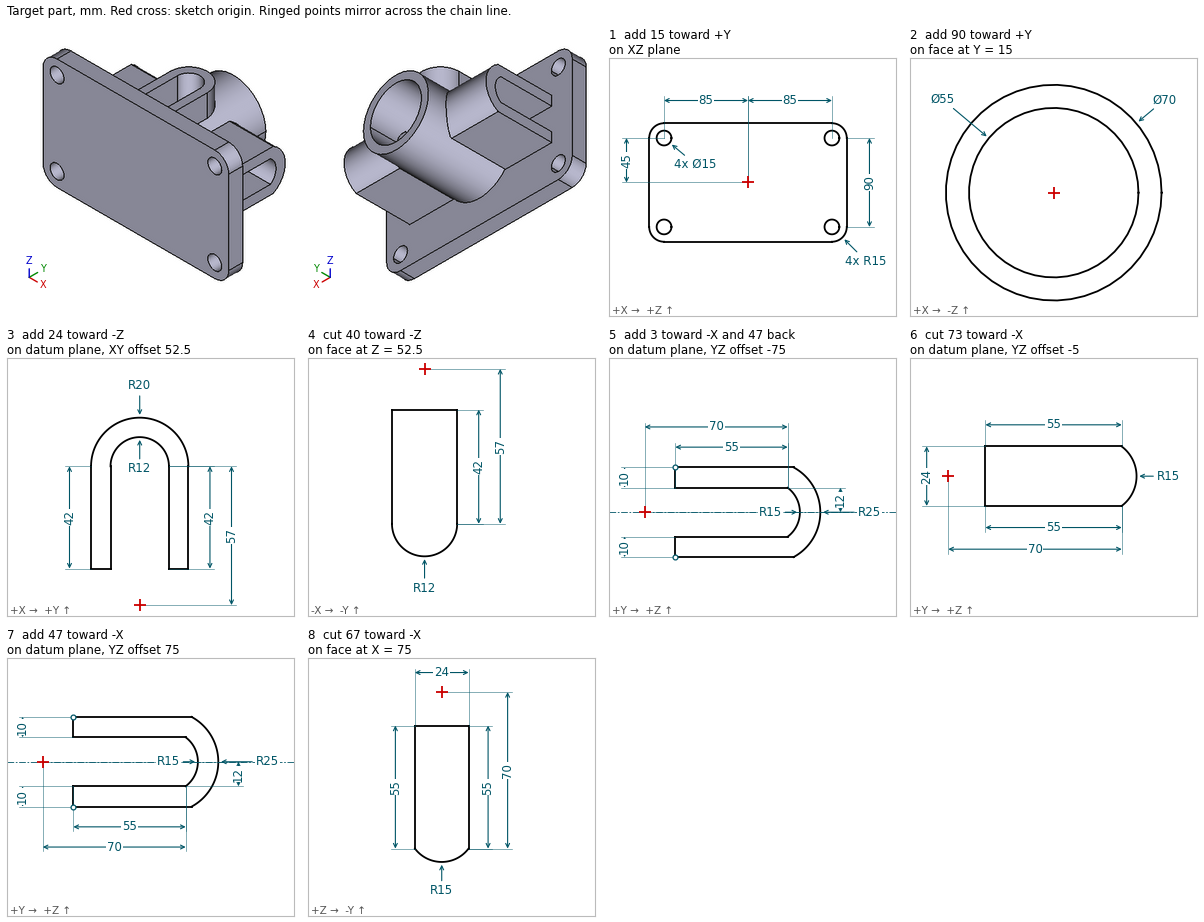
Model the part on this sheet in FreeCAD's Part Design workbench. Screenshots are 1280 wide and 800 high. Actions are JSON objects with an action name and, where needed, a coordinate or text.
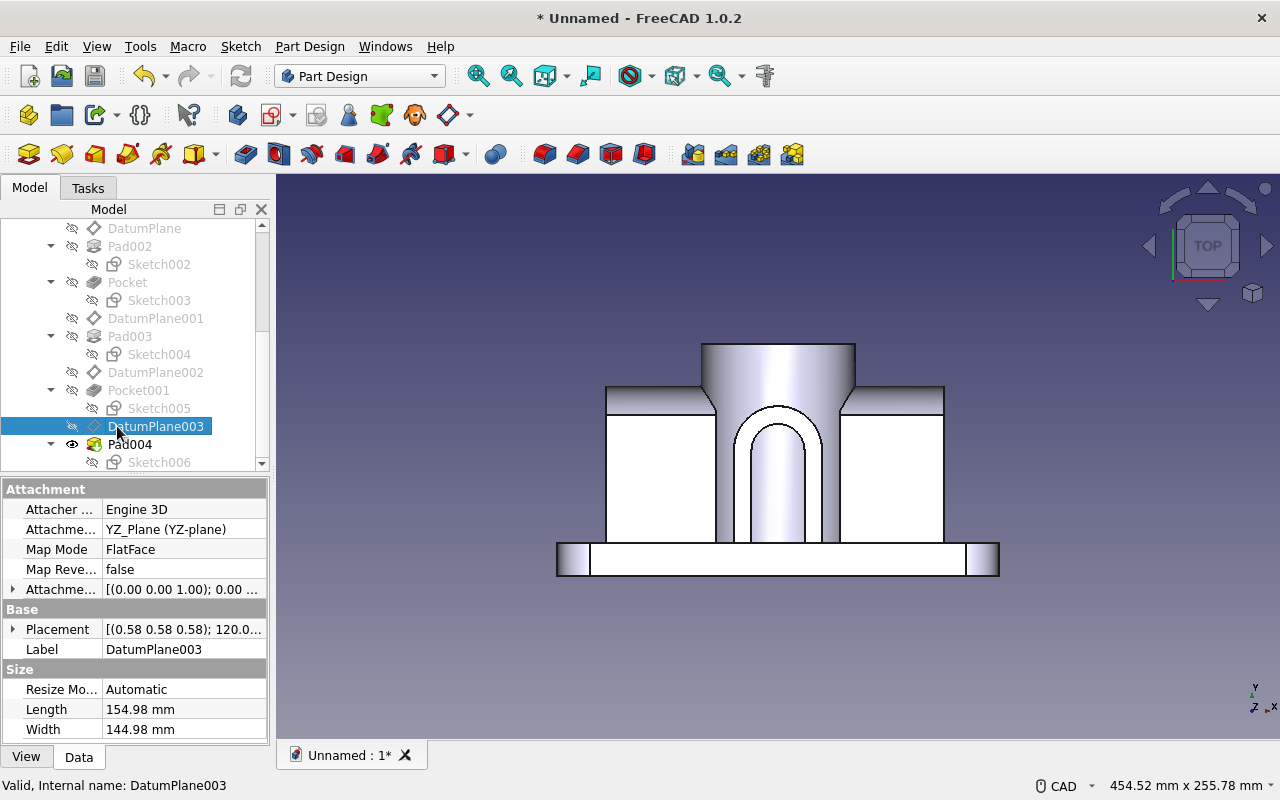
{"action": "left_click", "coordinate": [479, 76]}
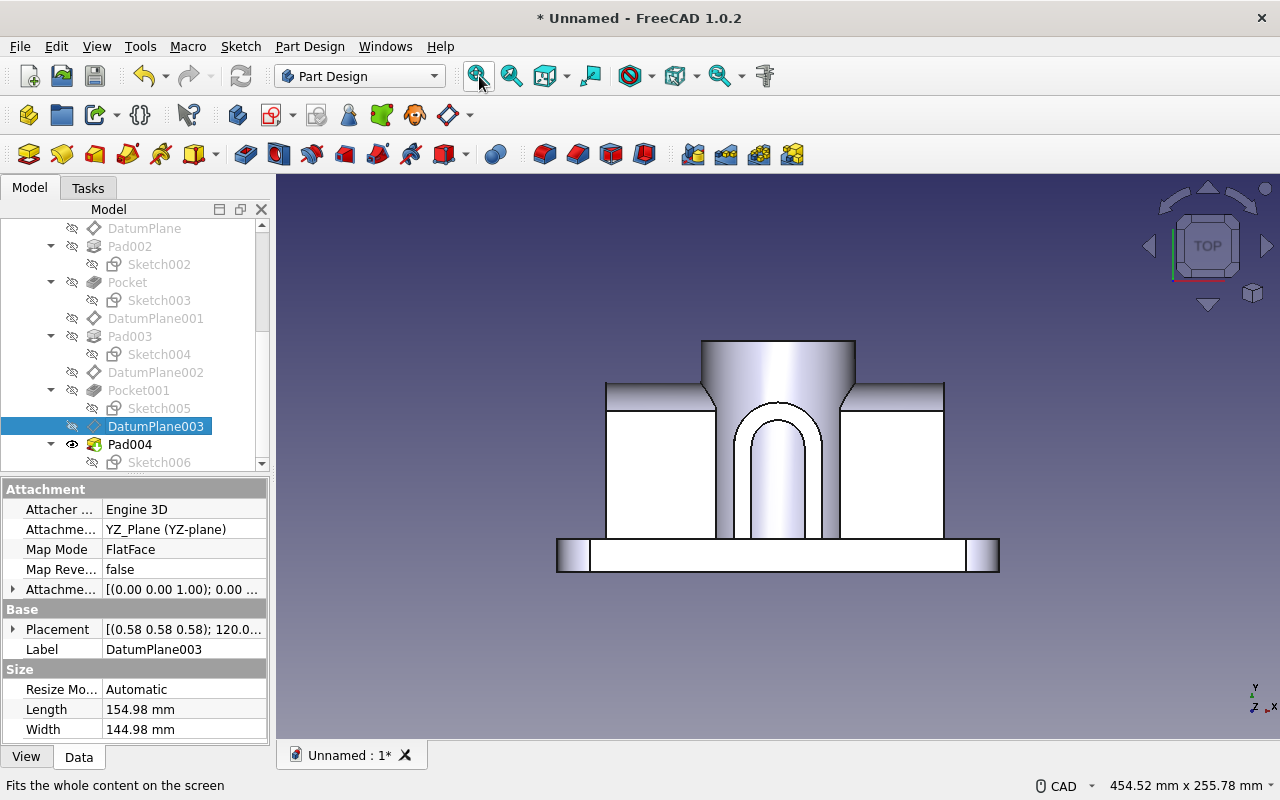
{"action": "key", "text": "0"}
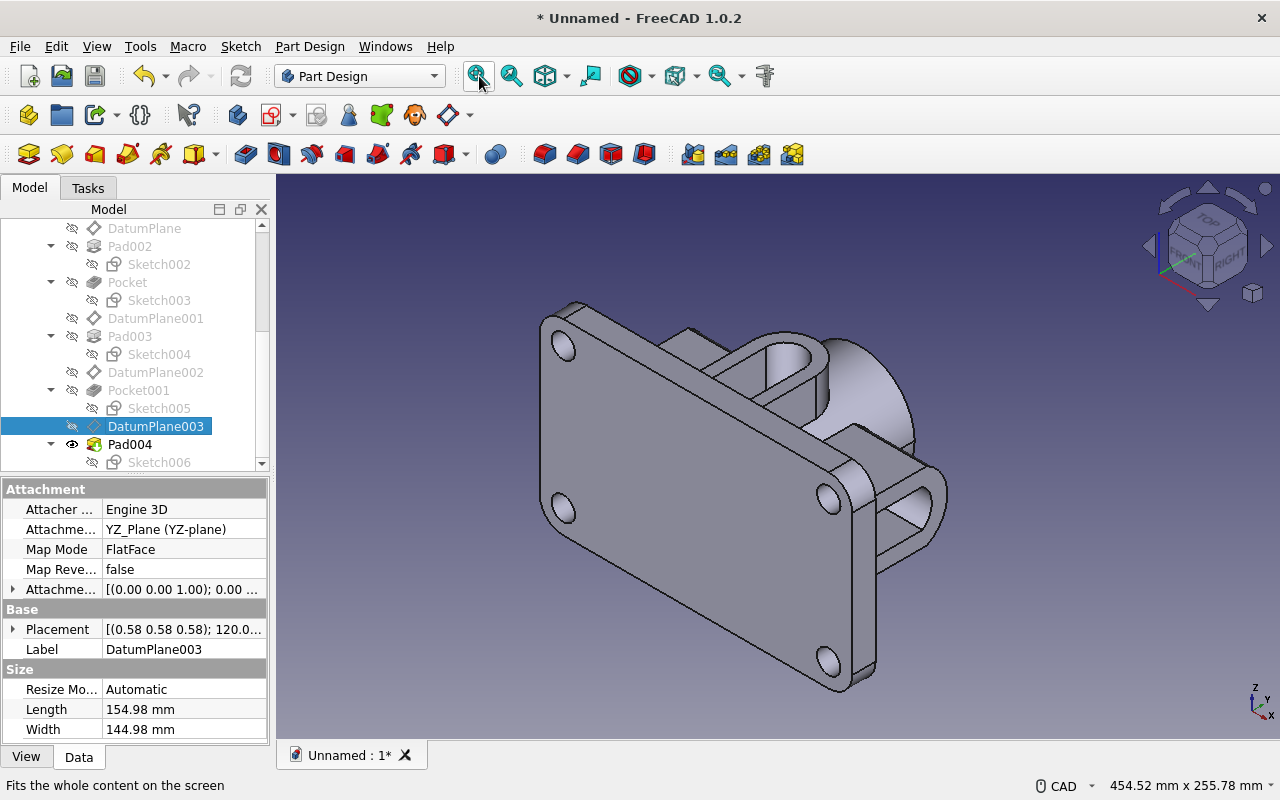
{"action": "left_click", "coordinate": [940, 497]}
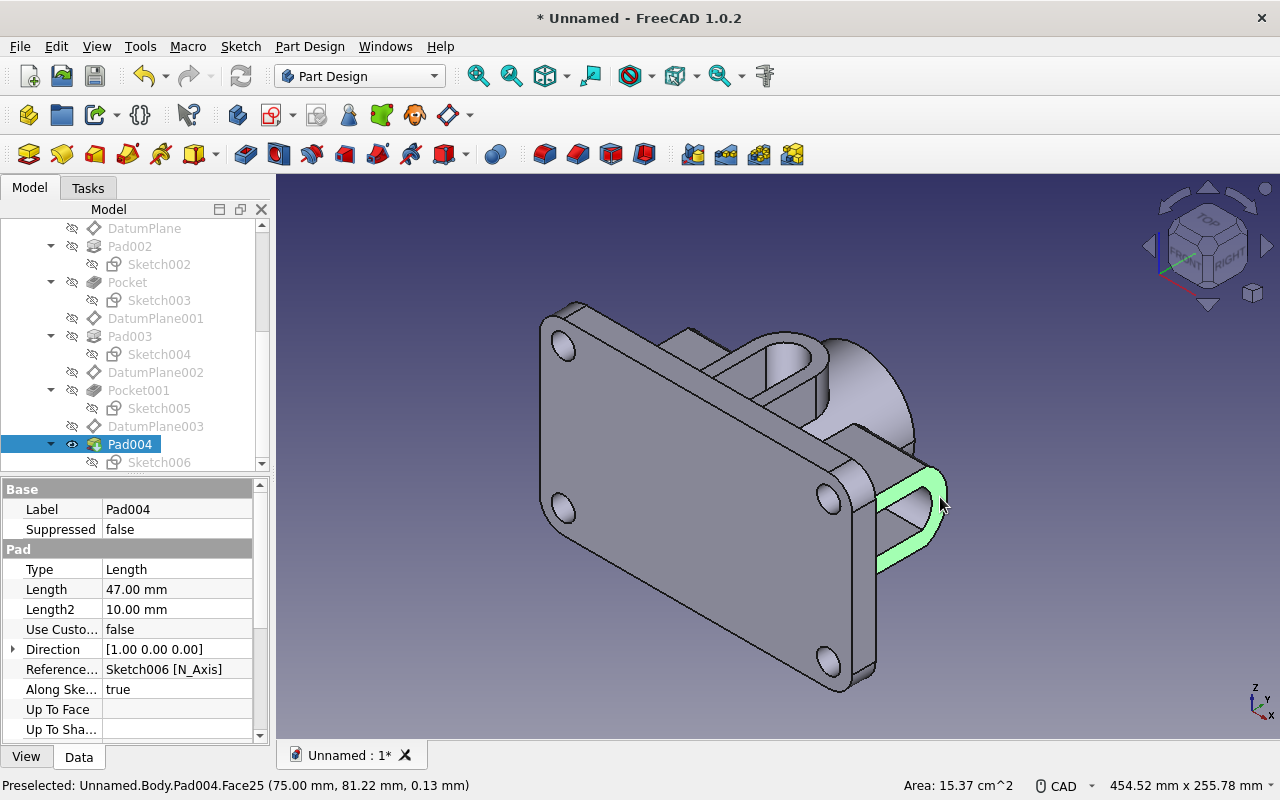
{"action": "left_click", "coordinate": [270, 116]}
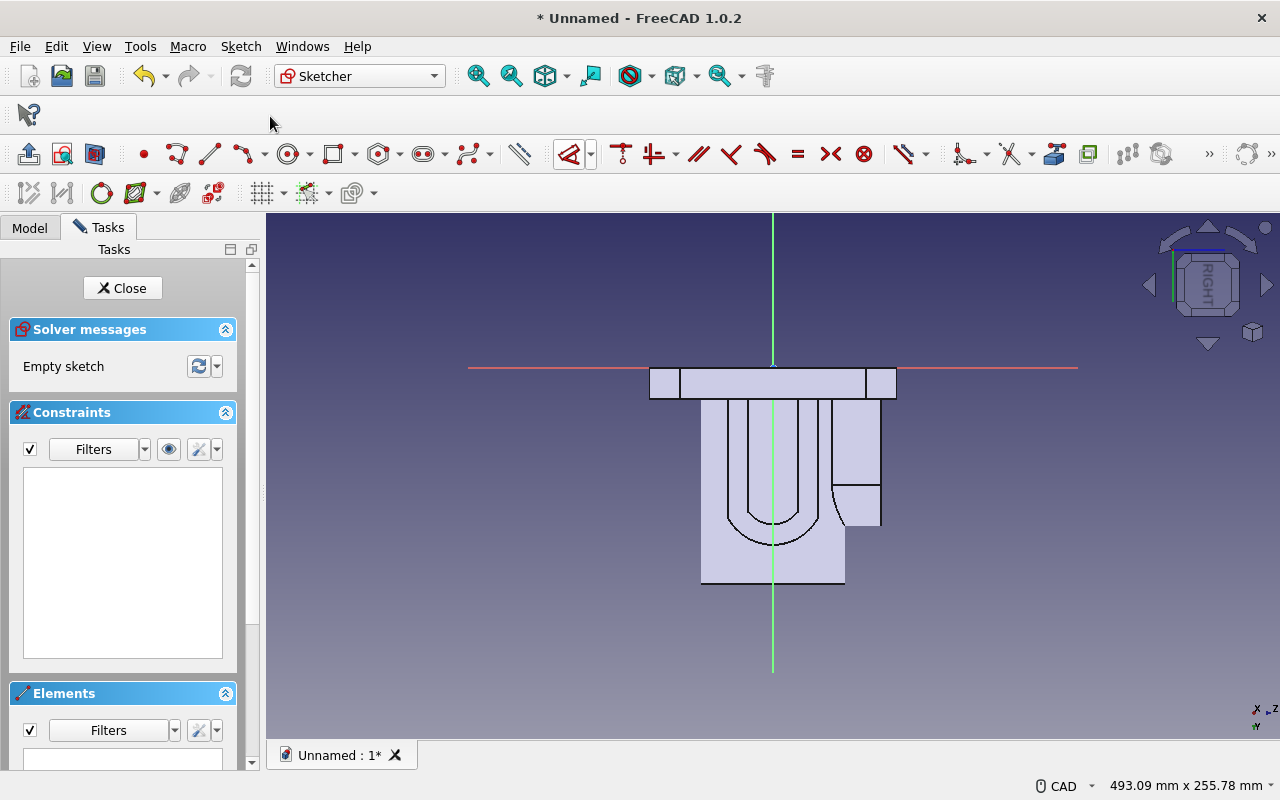
{"action": "left_click", "coordinate": [95, 154]}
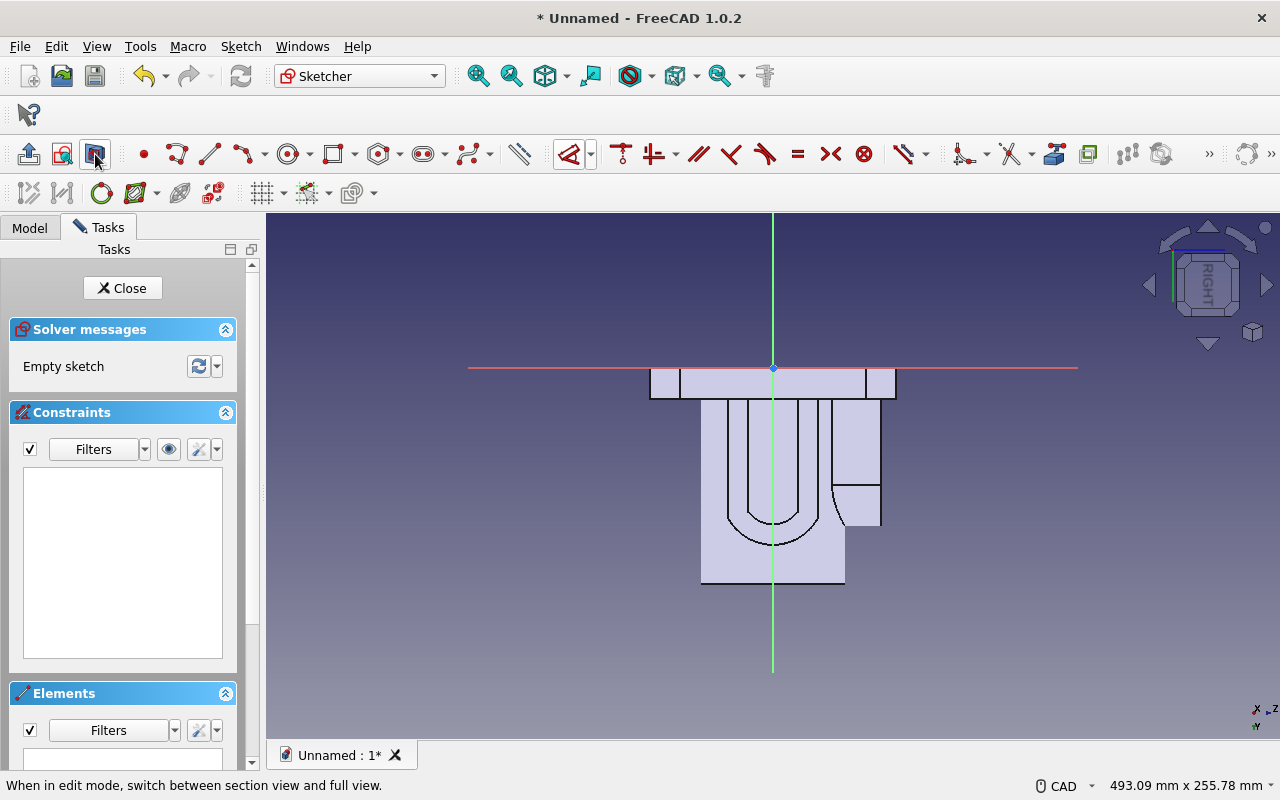
{"action": "scroll", "coordinate": [829, 422], "scroll_direction": "up", "scroll_amount": 4}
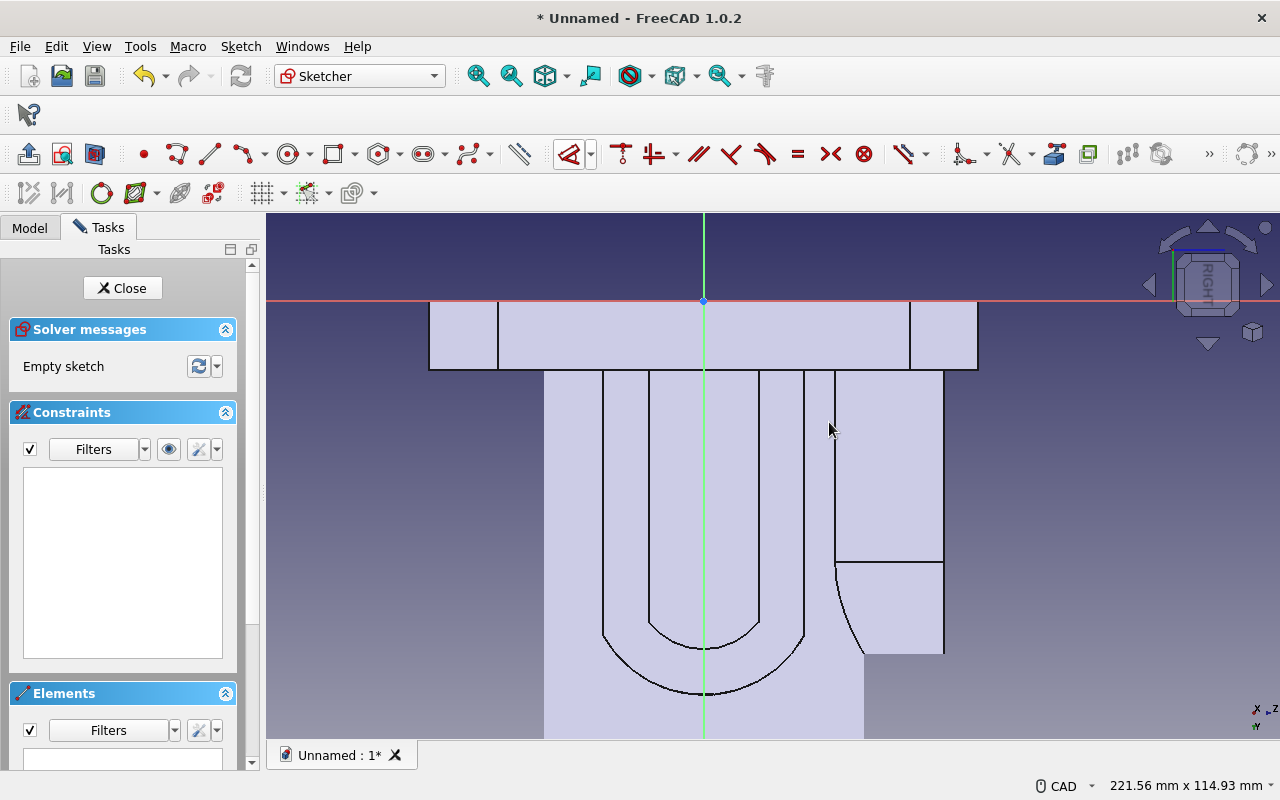
{"action": "key", "text": "g m"}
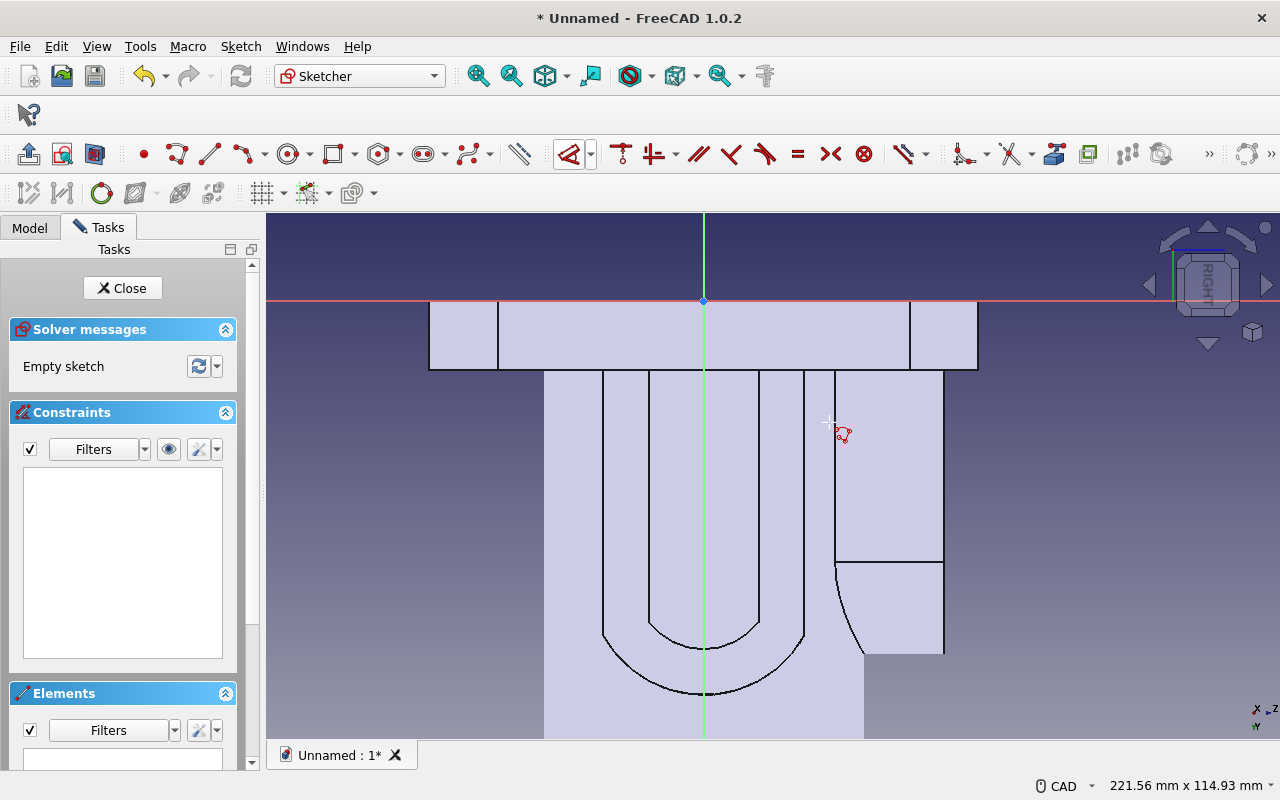
{"action": "left_click", "coordinate": [759, 622]}
{"action": "left_click", "coordinate": [759, 370]}
{"action": "left_click", "coordinate": [649, 370]}
{"action": "left_click", "coordinate": [649, 622]}
{"action": "right_click", "coordinate": [649, 622]}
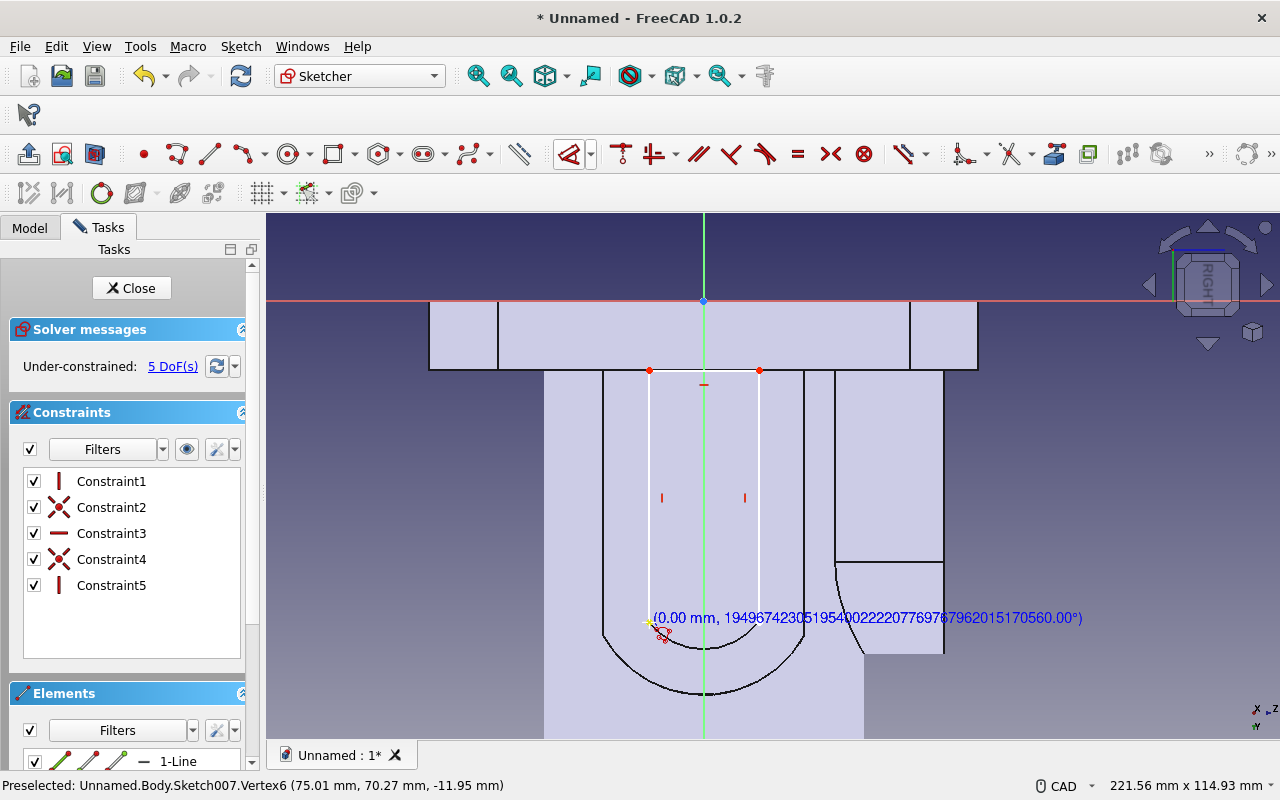
{"action": "left_click", "coordinate": [242, 154]}